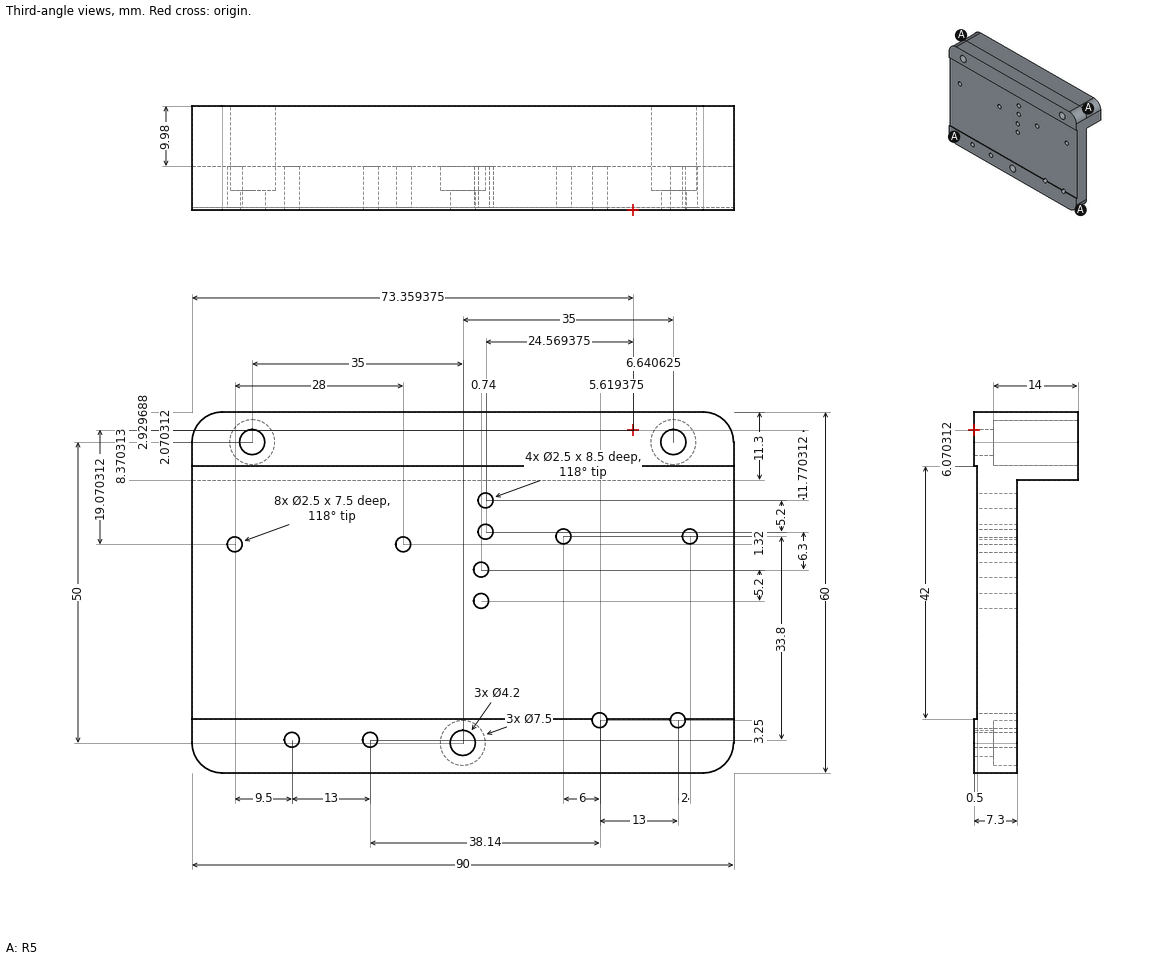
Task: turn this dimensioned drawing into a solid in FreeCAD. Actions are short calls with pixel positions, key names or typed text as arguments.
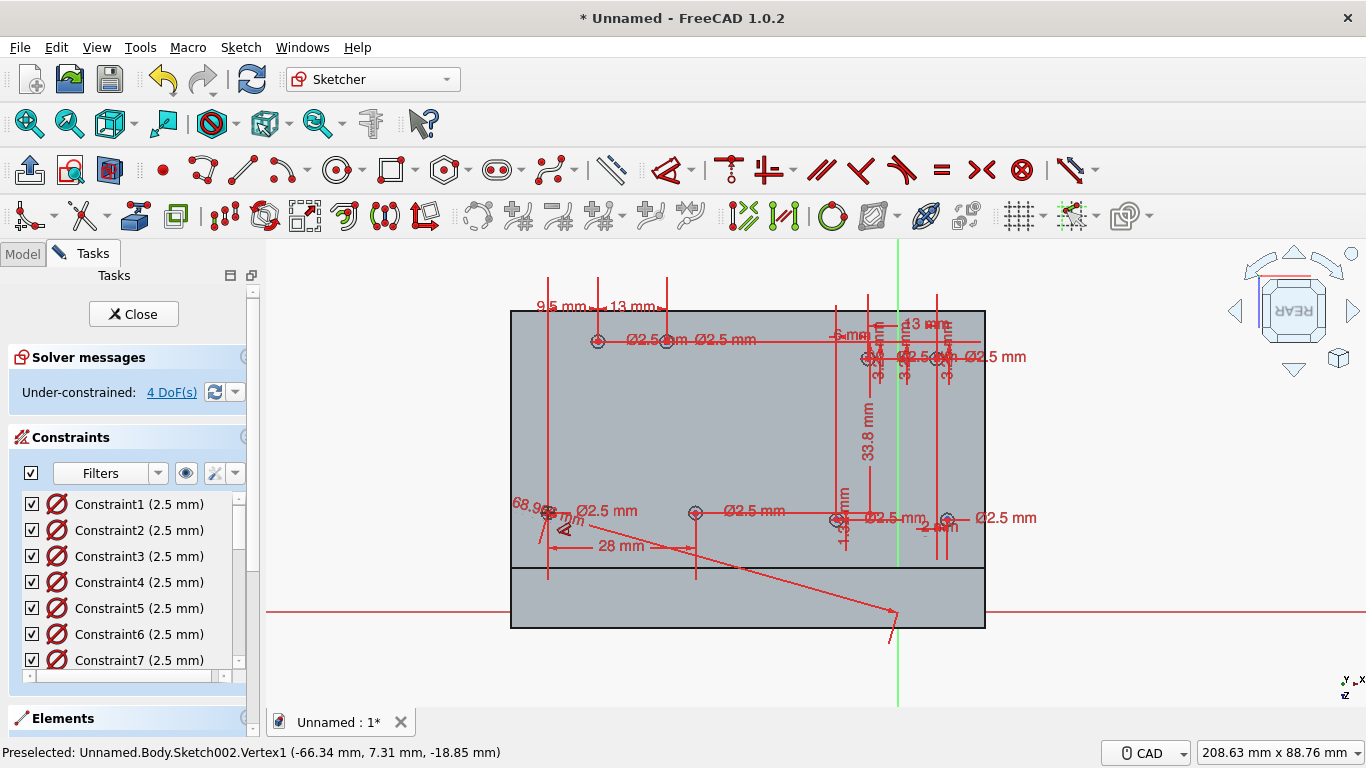
scroll(836, 520, up, 9)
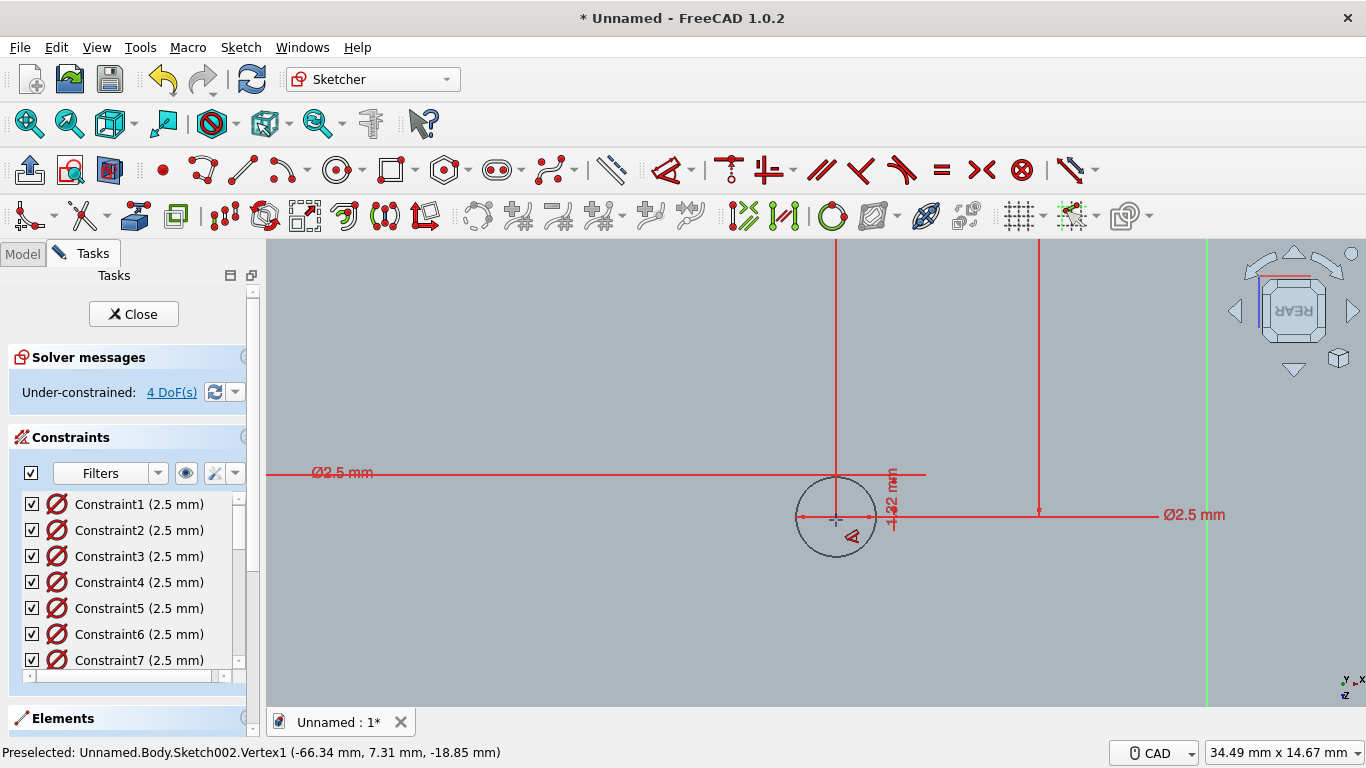
click(836, 517)
click(966, 496)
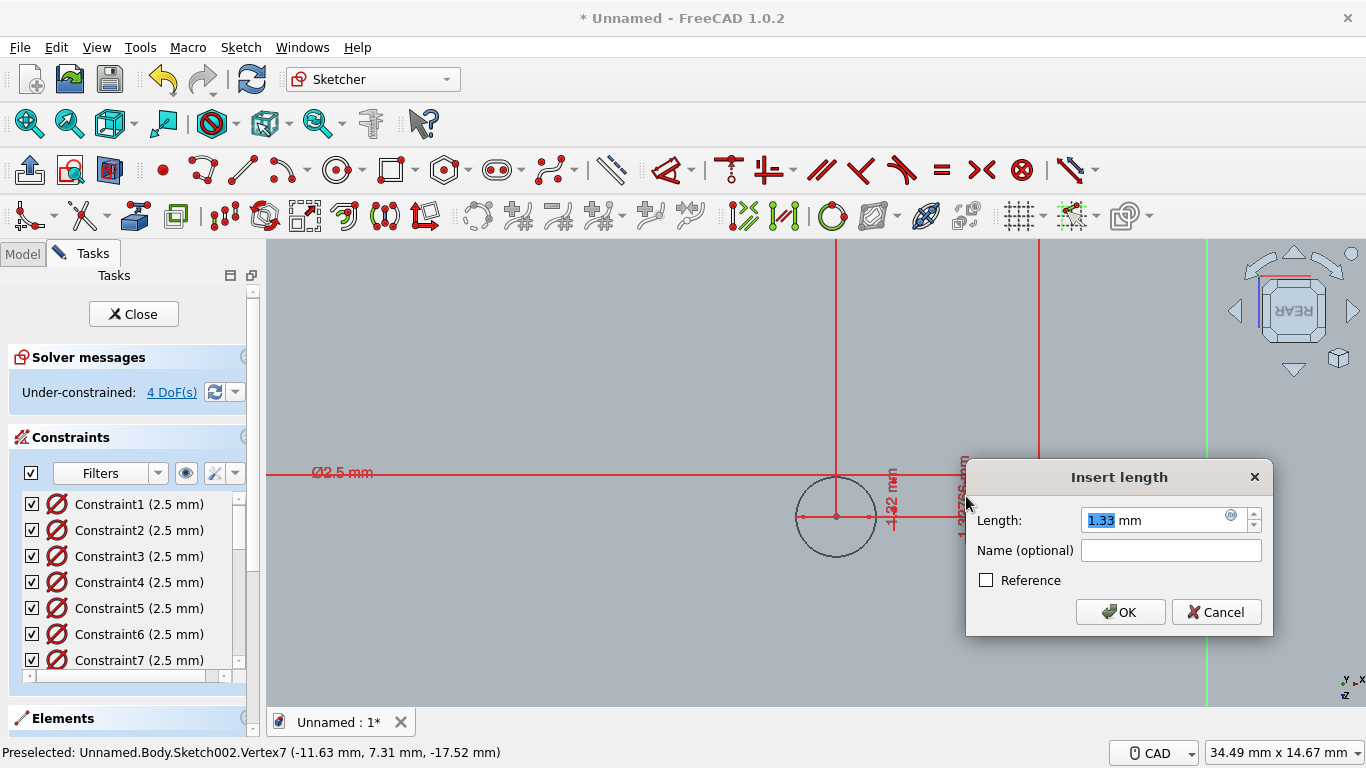
text(1.32)
key(Return)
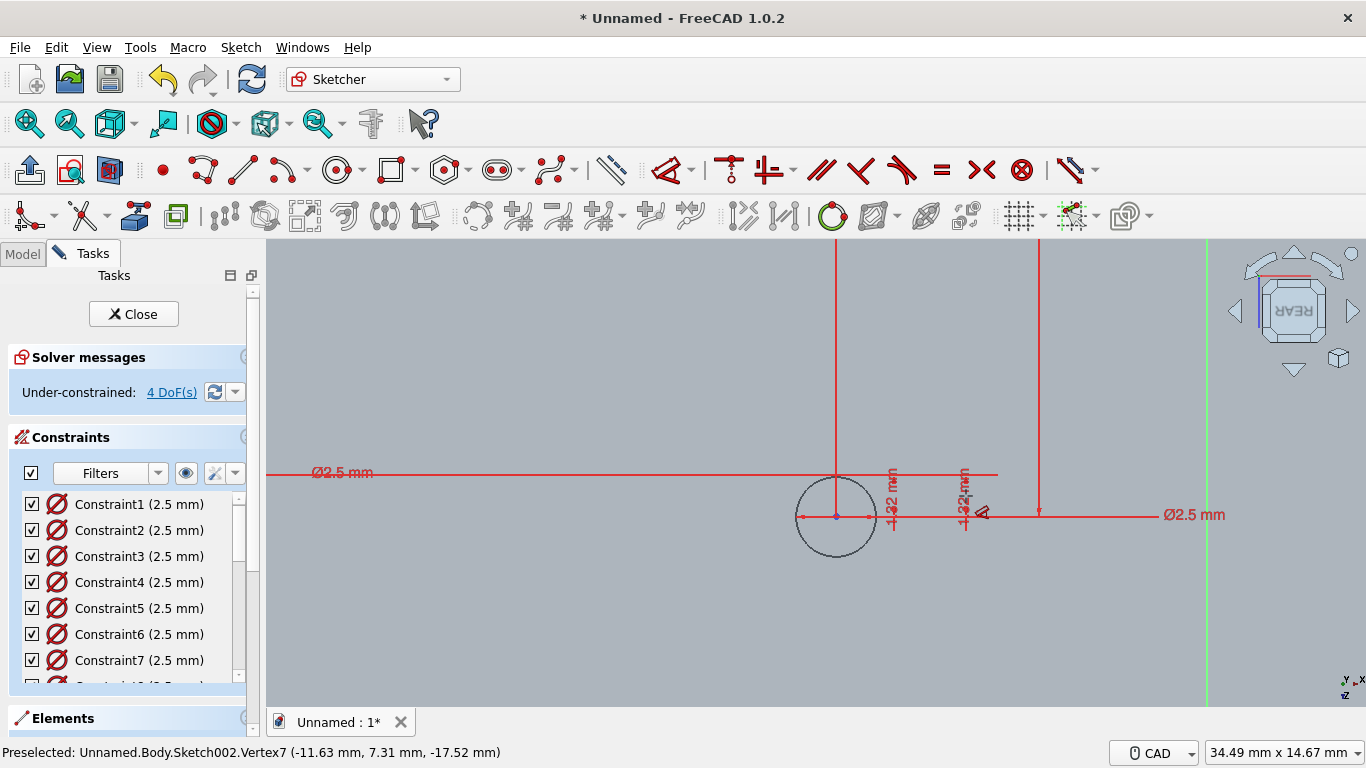
scroll(836, 520, down, 9)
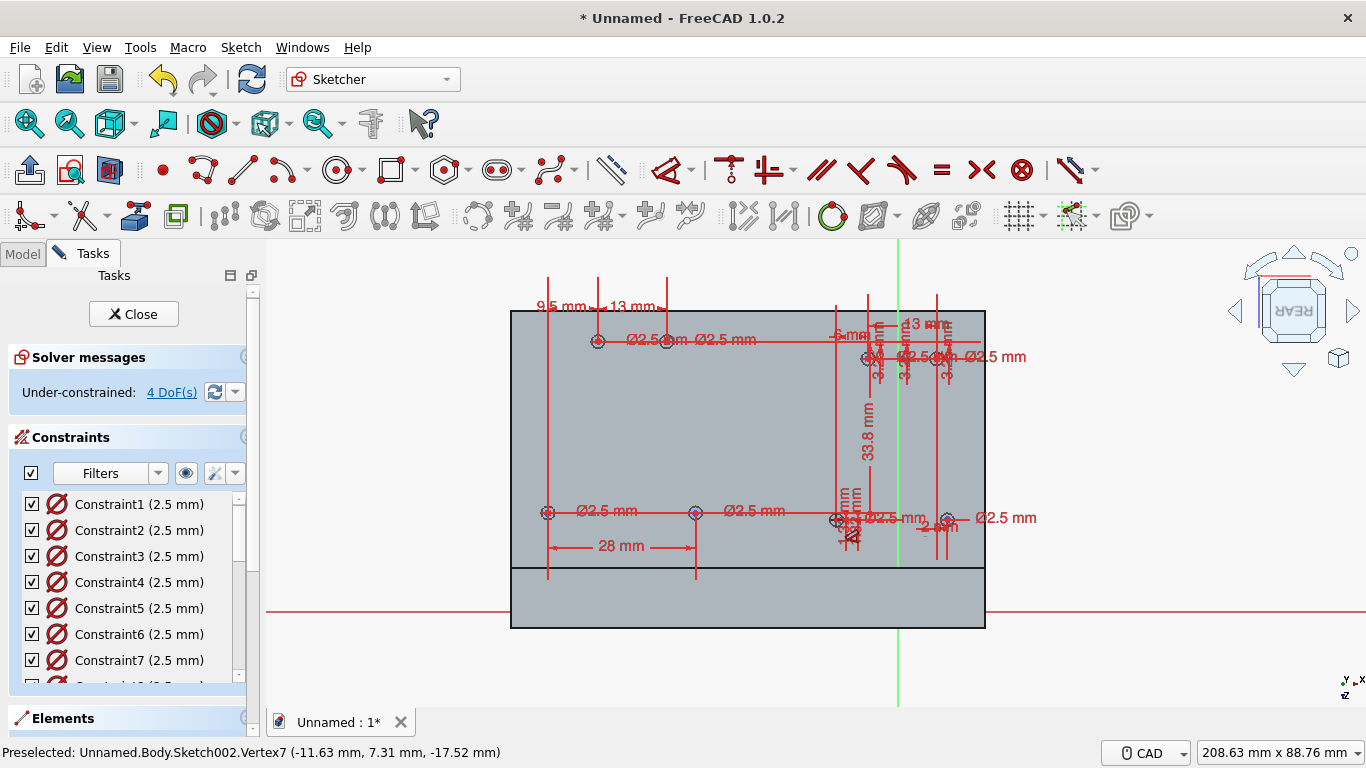
scroll(696, 513, up, 9)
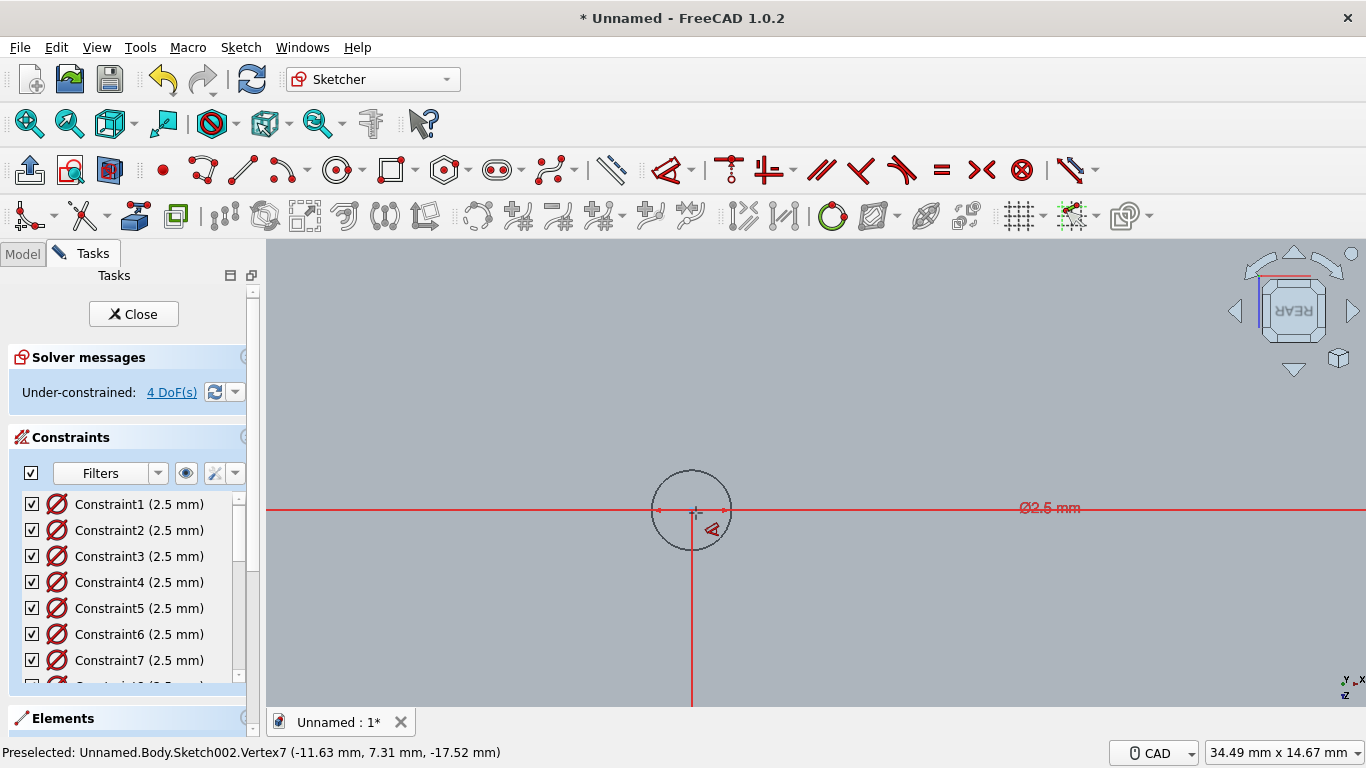
click(692, 510)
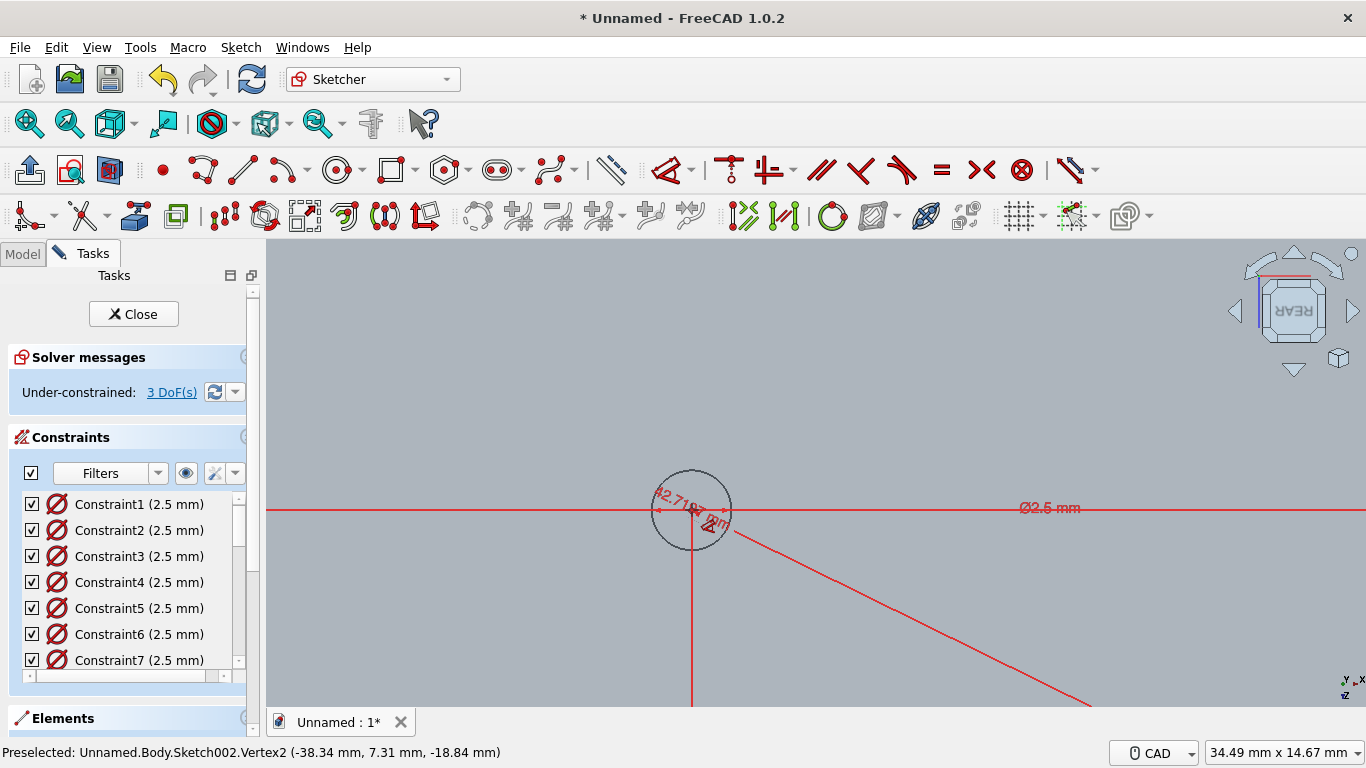
scroll(696, 513, down, 9)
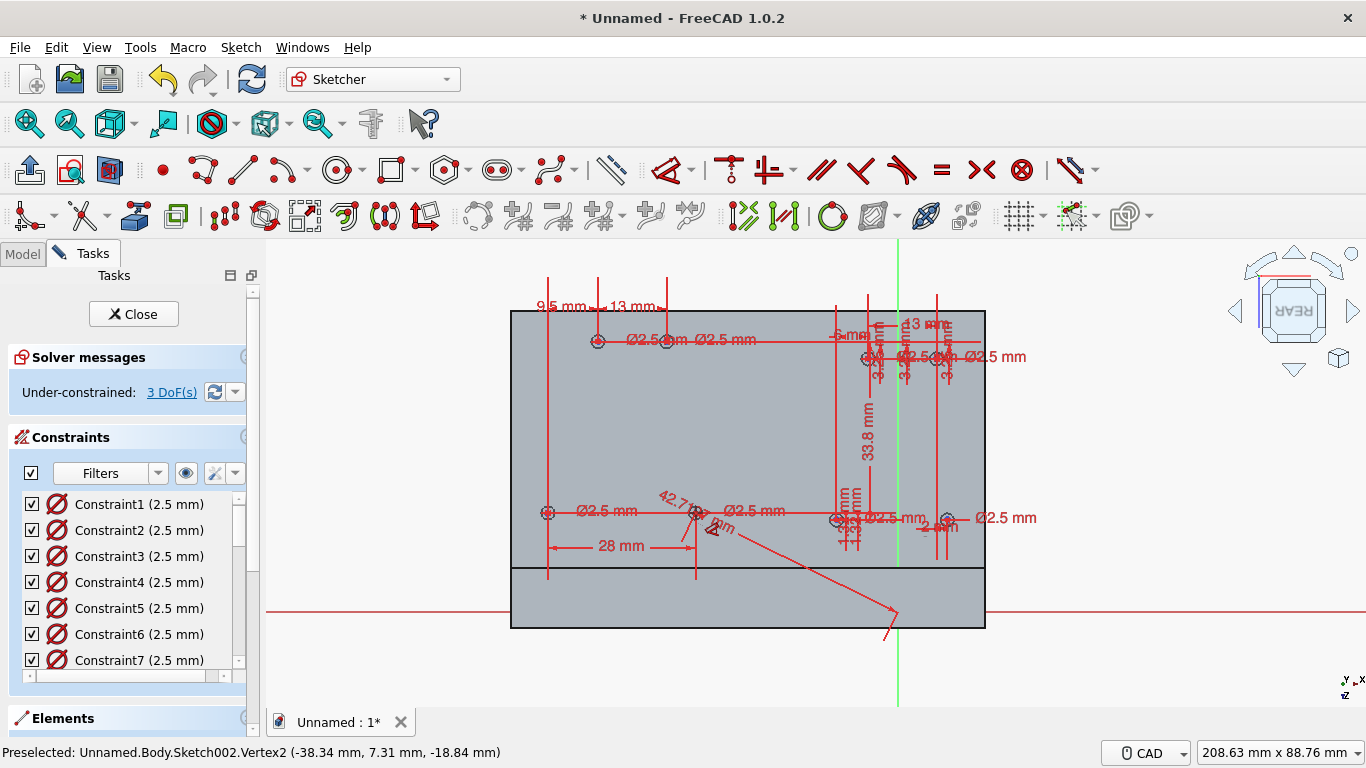
scroll(947, 520, up, 9)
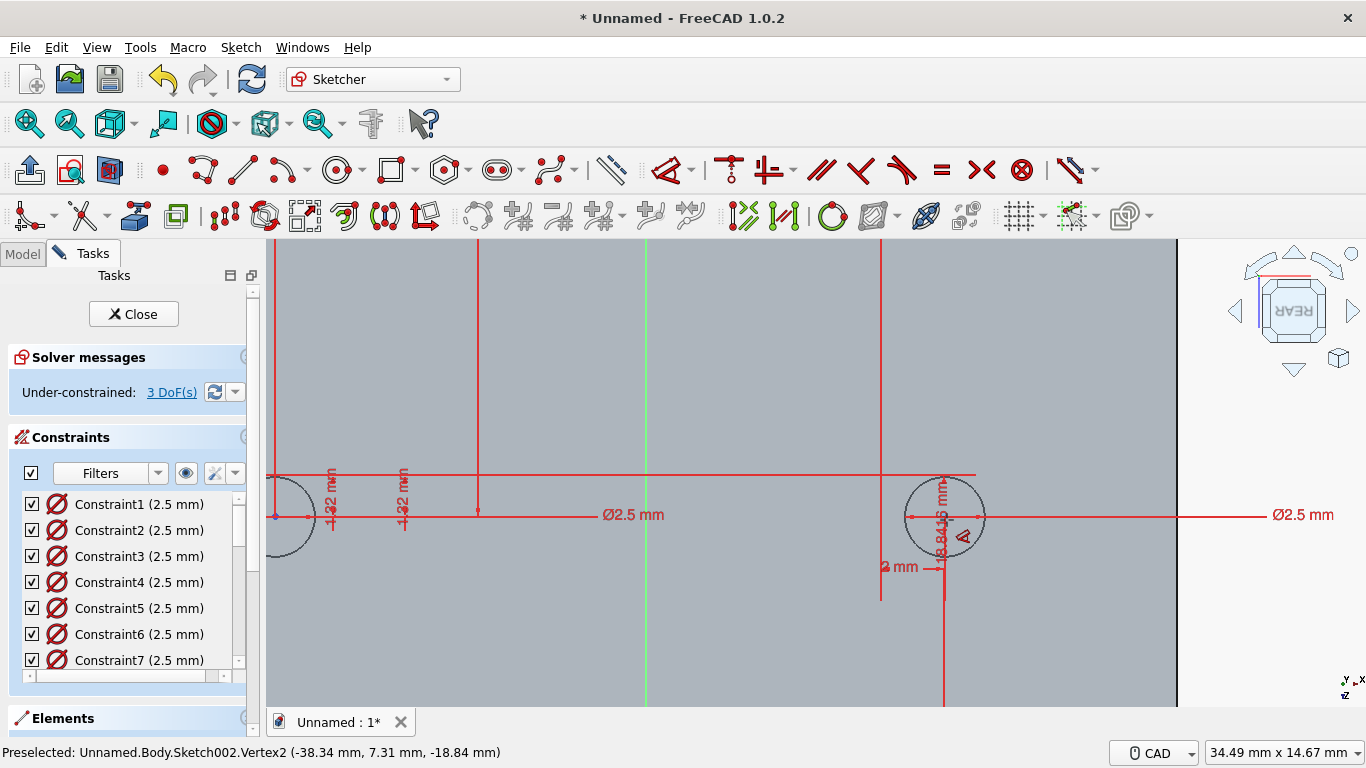
click(945, 517)
click(1003, 496)